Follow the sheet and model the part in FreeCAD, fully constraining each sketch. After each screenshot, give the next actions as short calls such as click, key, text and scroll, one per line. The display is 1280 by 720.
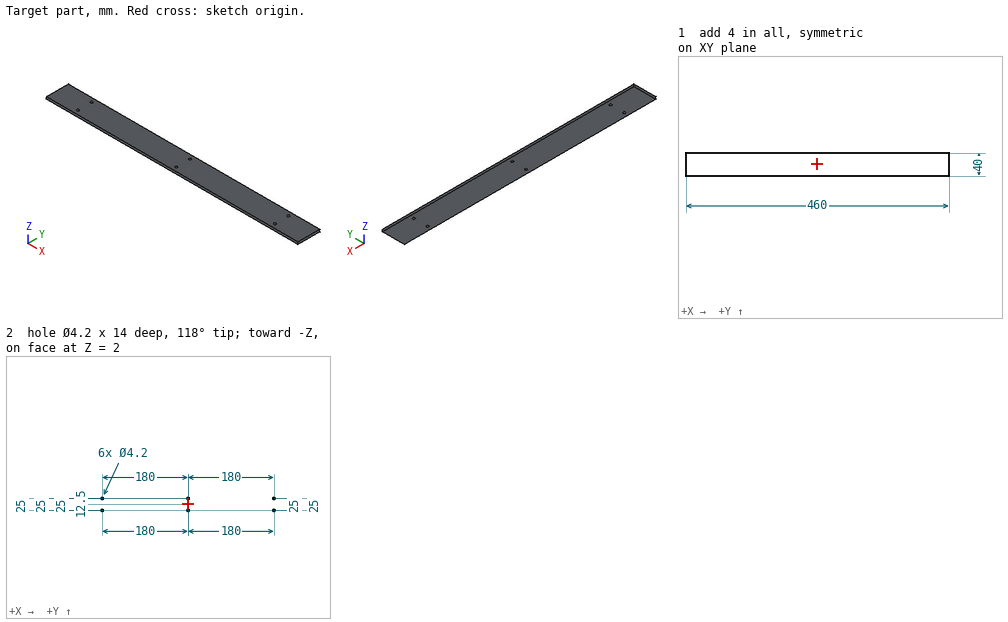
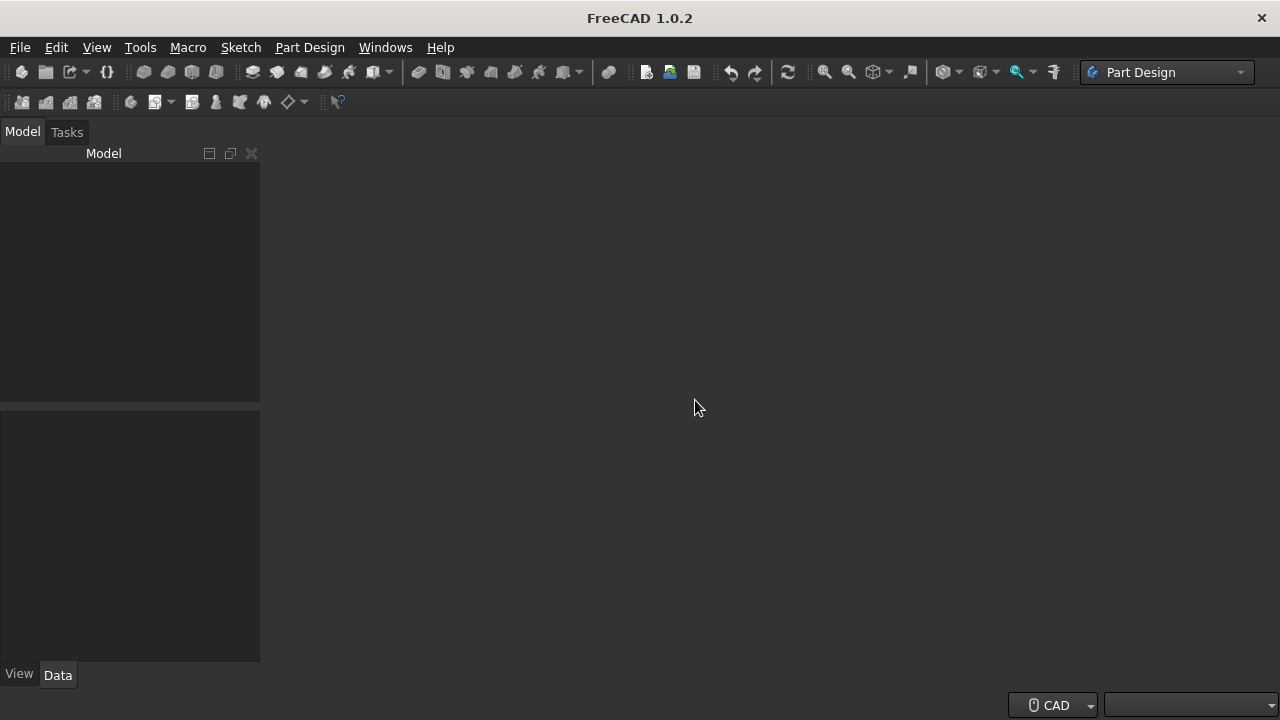
key(ctrl+n)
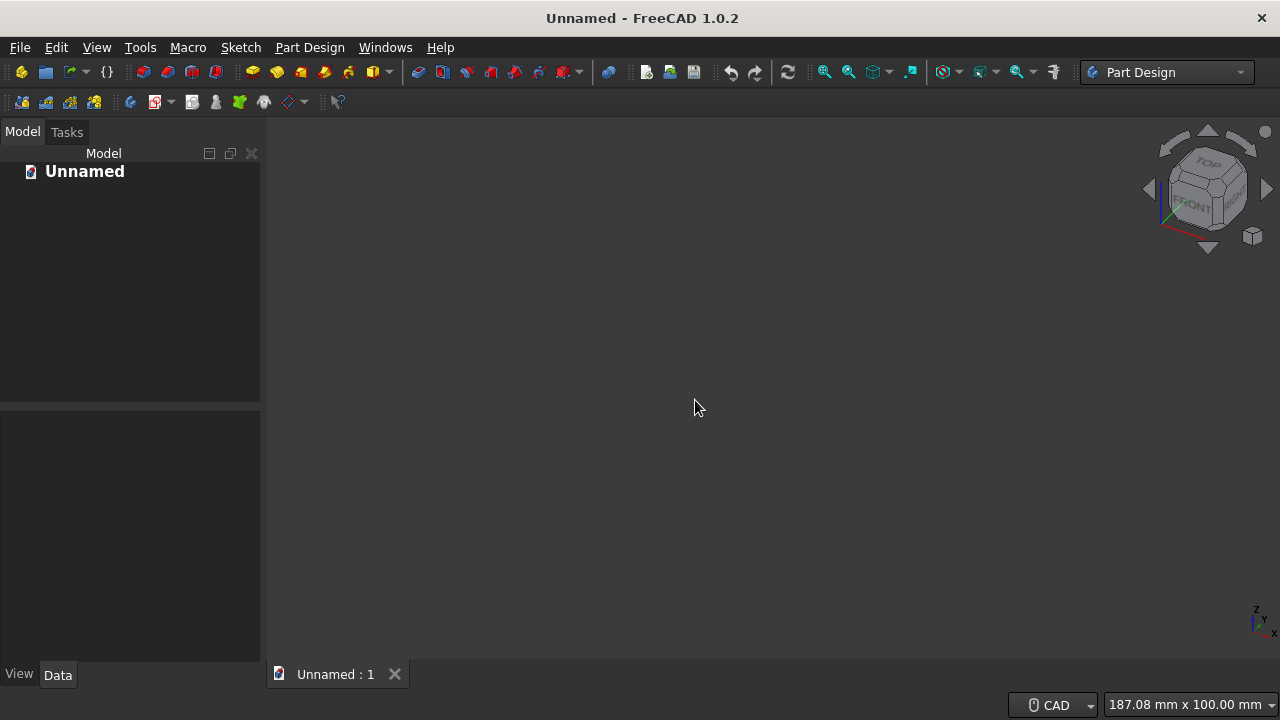
click(156, 102)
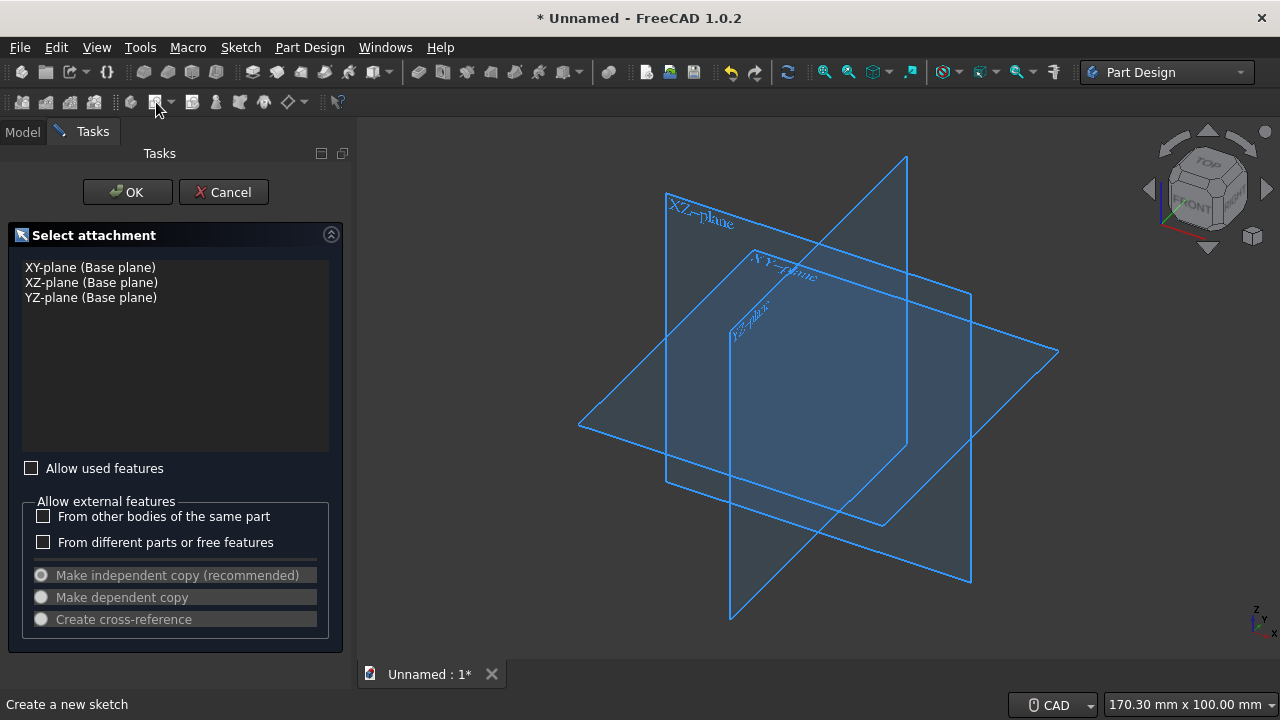
click(82, 268)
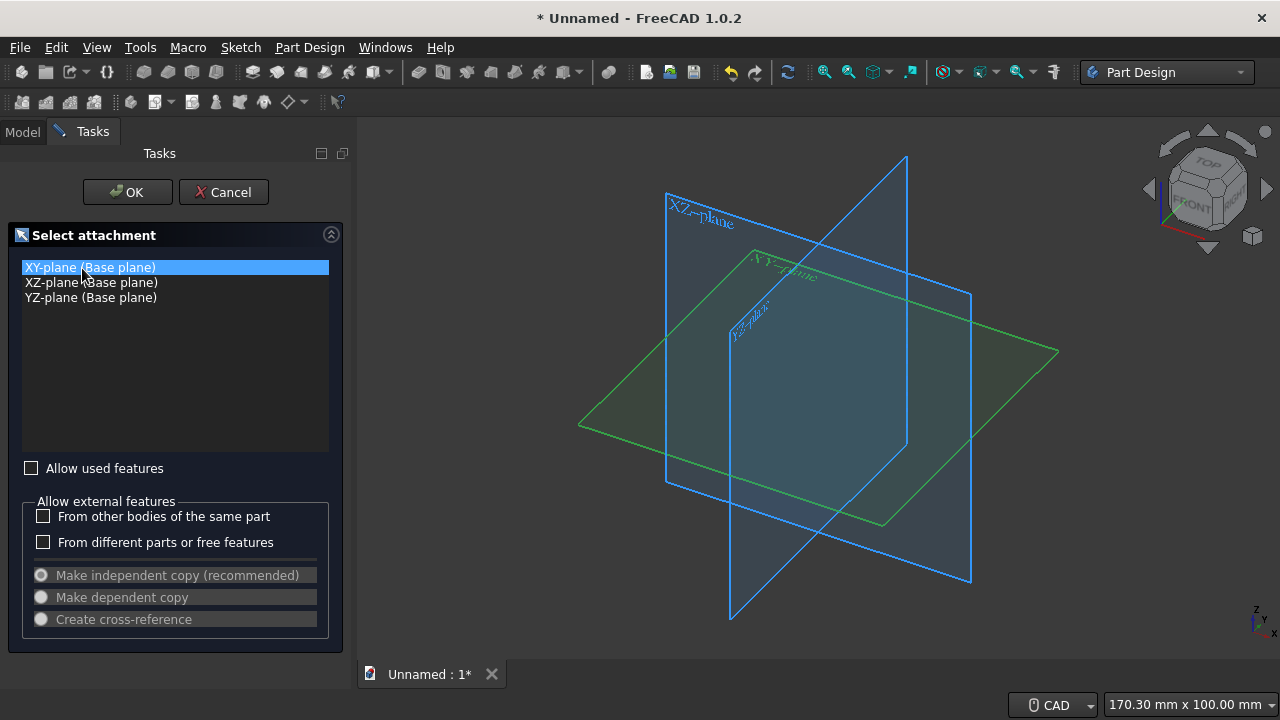
click(128, 192)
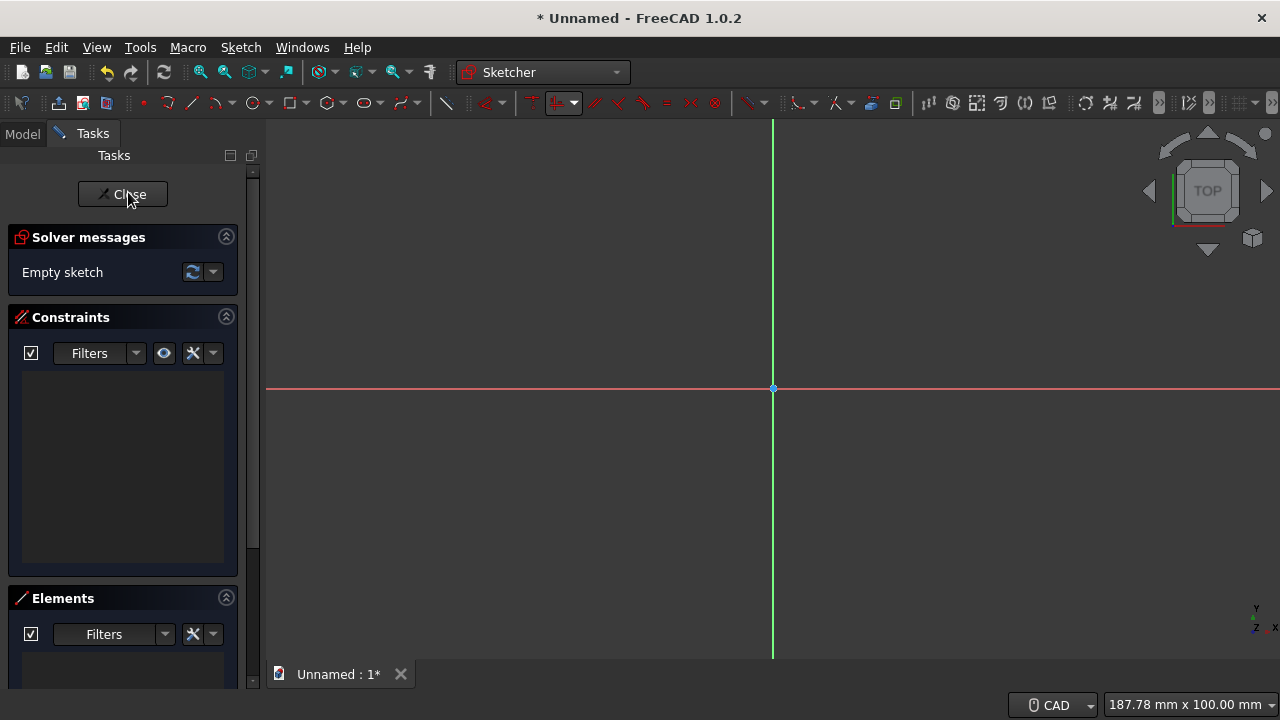
scroll(682, 389, down, 7)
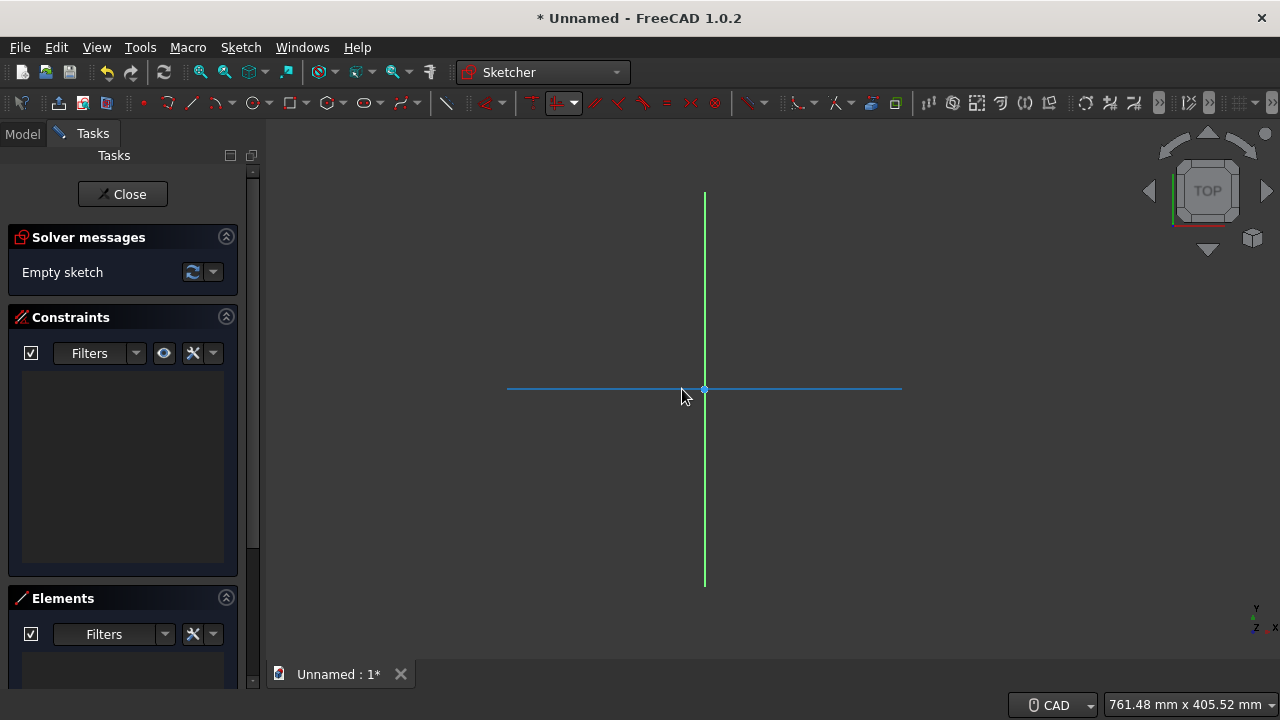
click(308, 104)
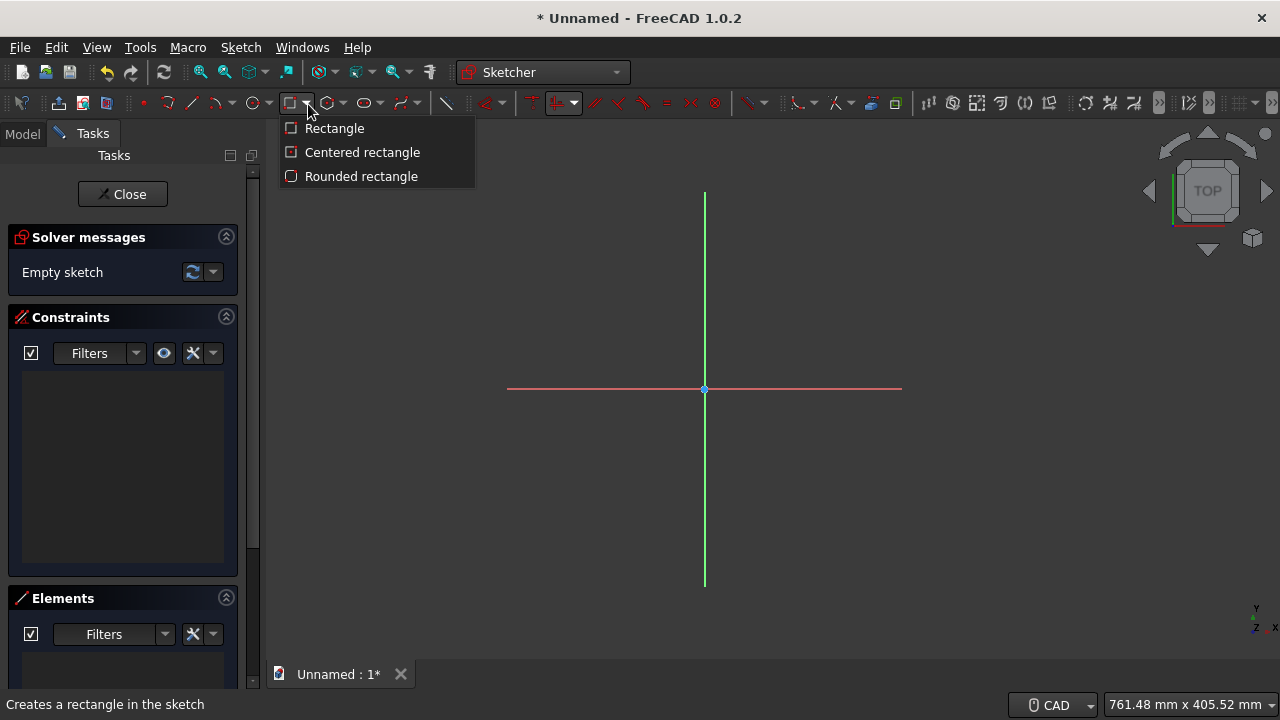
click(378, 152)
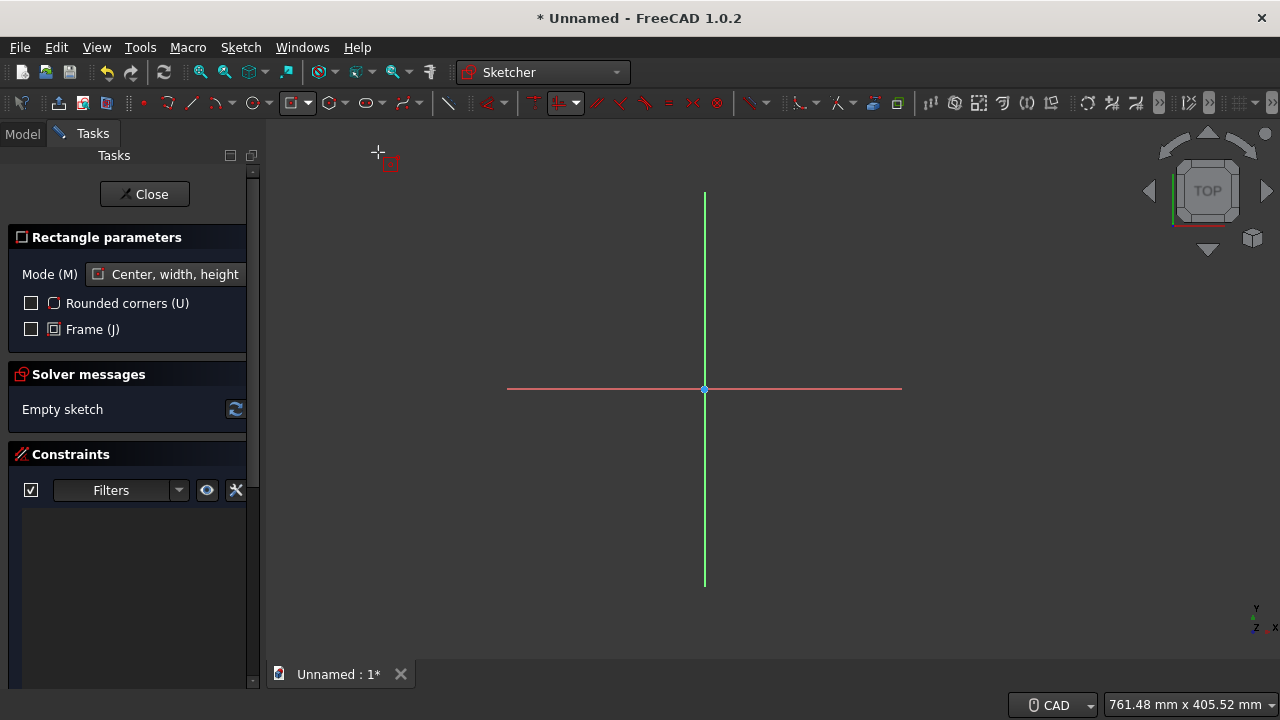
click(705, 389)
click(1011, 363)
key(Escape)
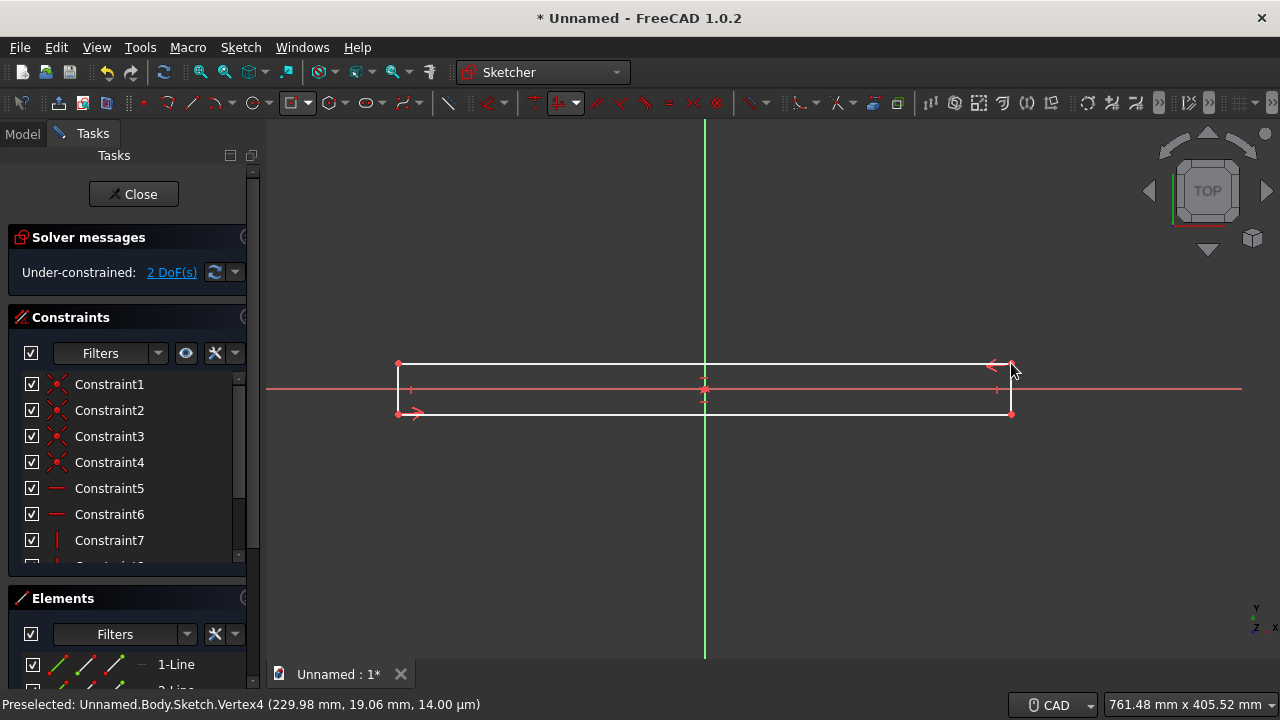
key(d)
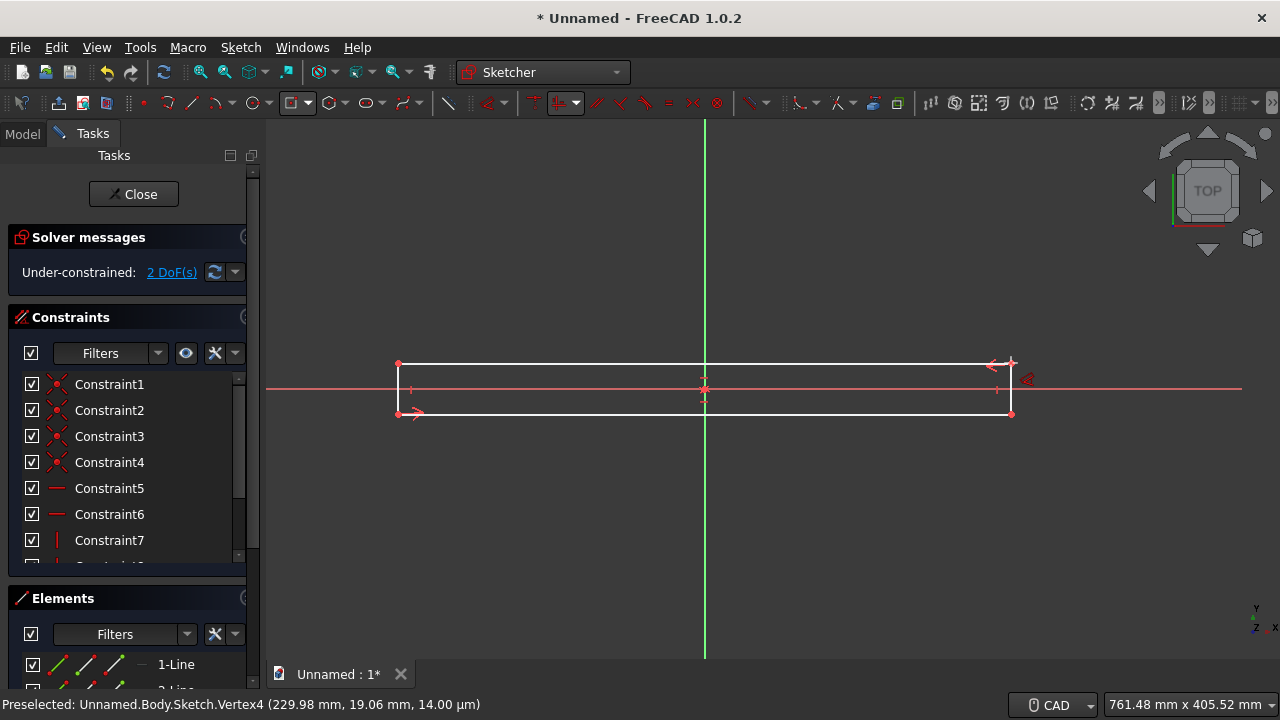
scroll(1011, 400, up, 2)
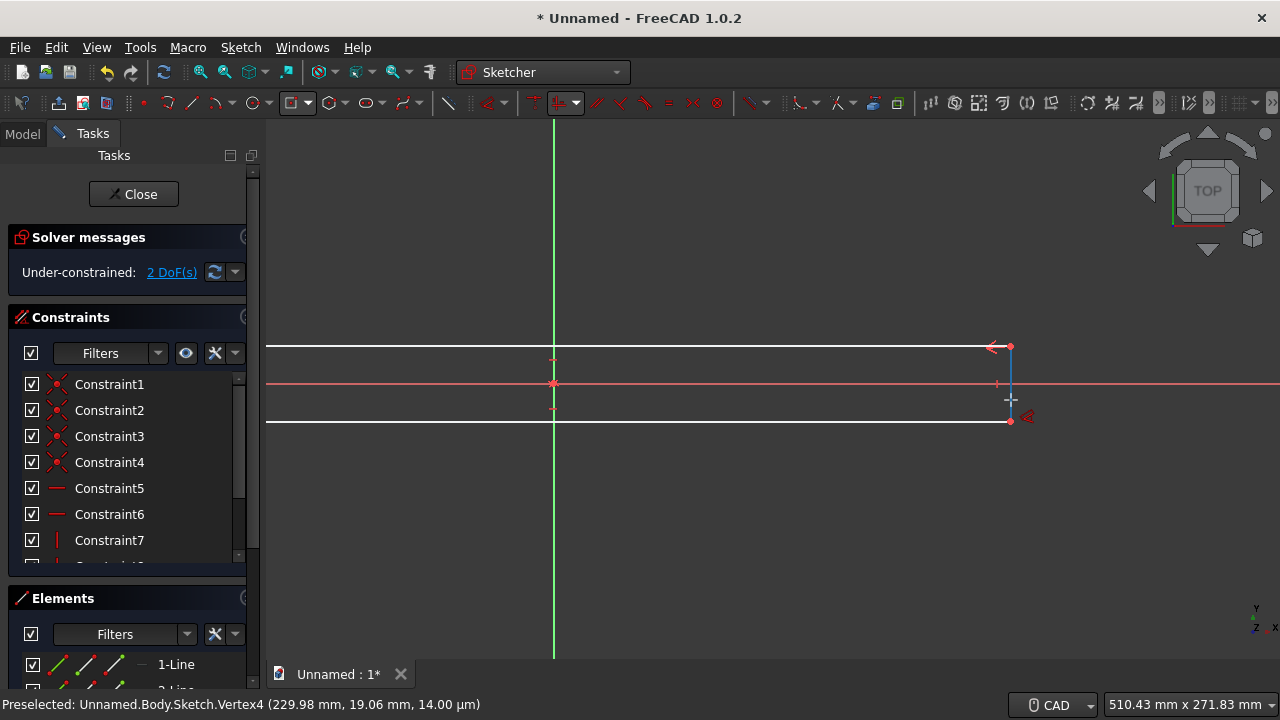
click(1011, 399)
click(1045, 366)